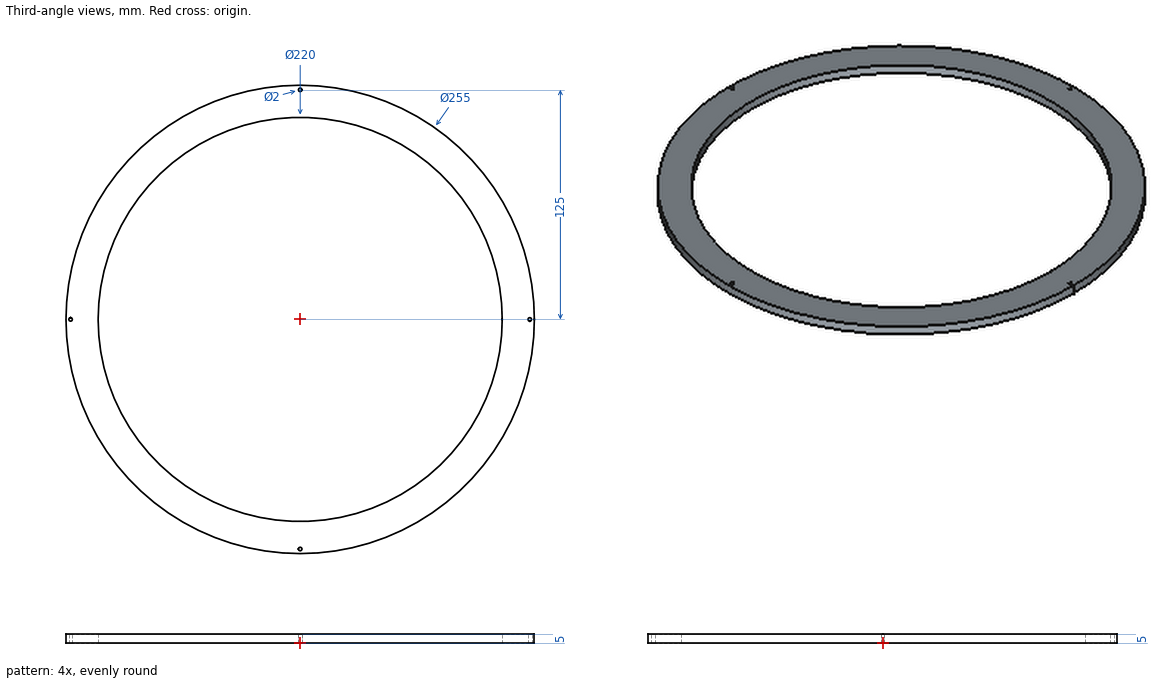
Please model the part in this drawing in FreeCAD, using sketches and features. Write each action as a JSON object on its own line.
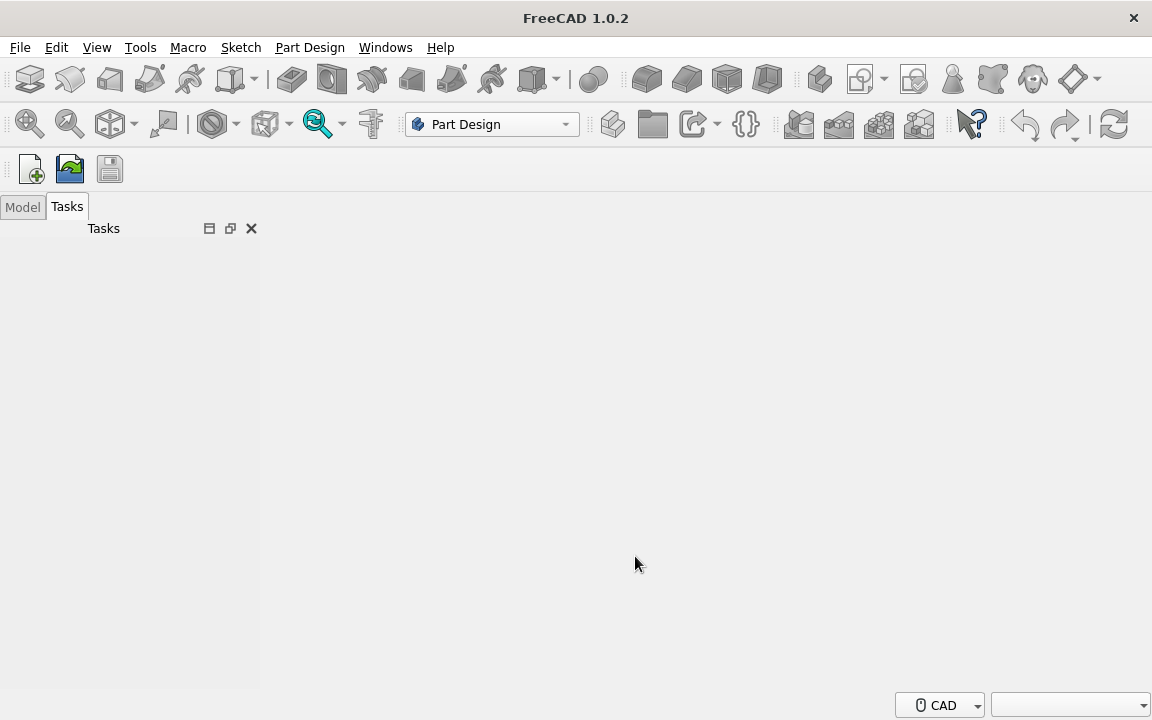
{"action": "left_click", "coordinate": [30, 170]}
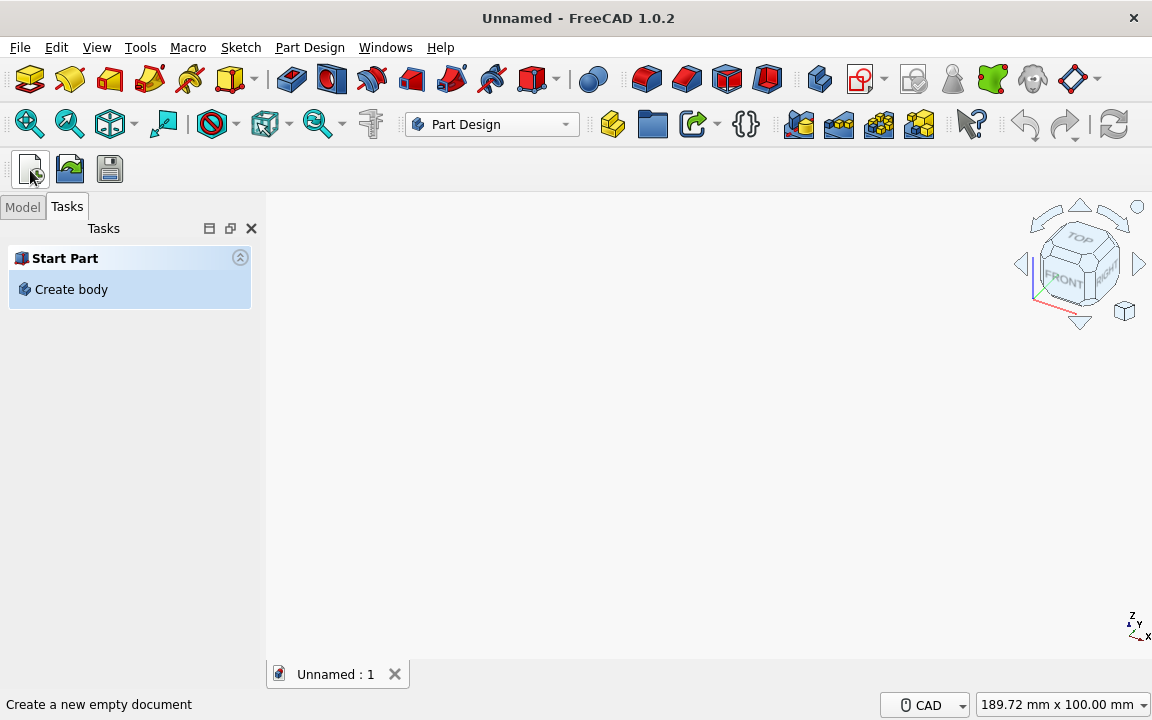
{"action": "left_click", "coordinate": [860, 80]}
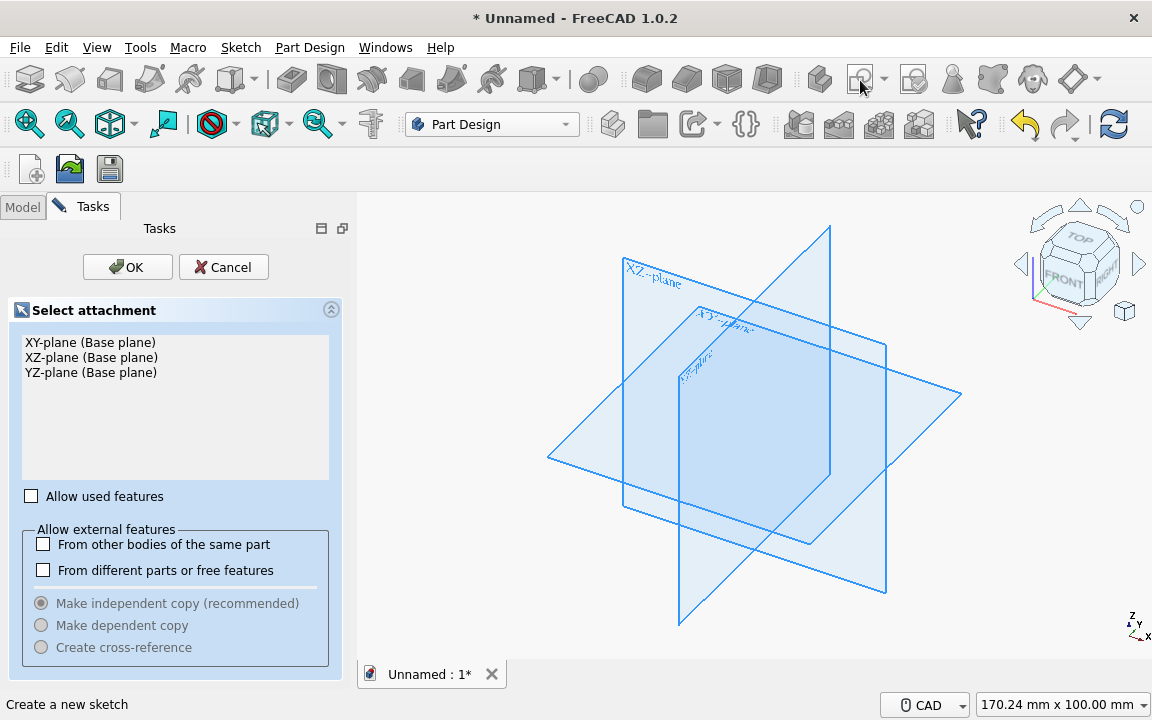
{"action": "left_click", "coordinate": [82, 342]}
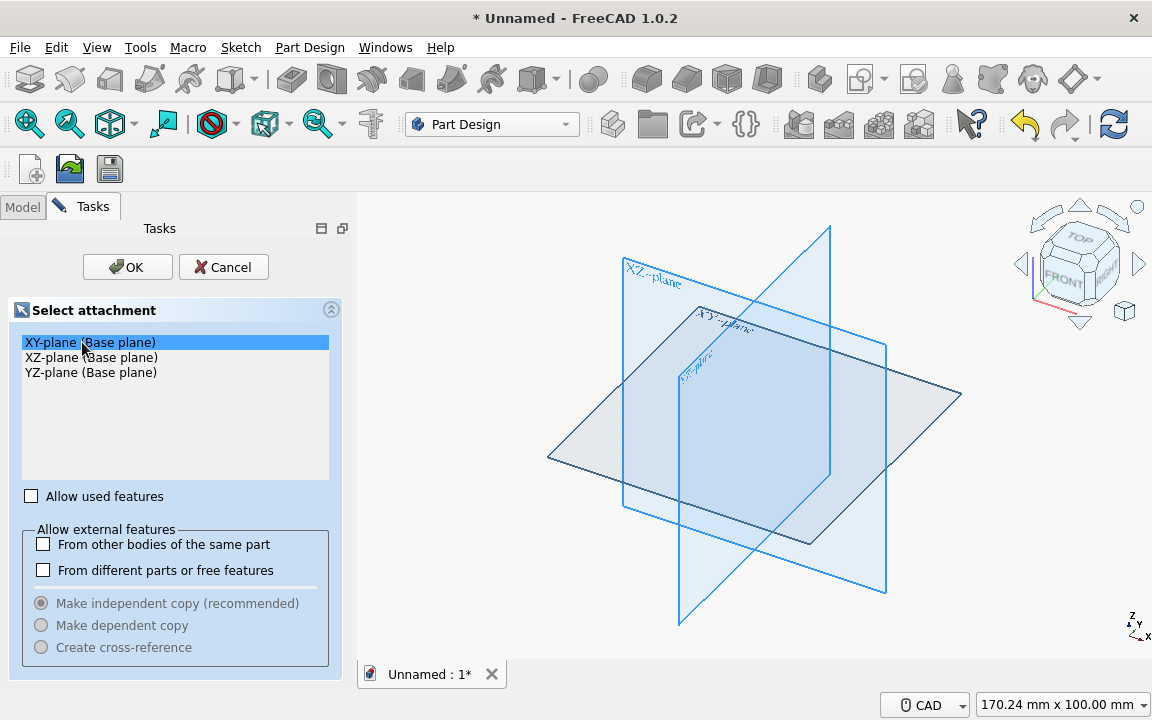
{"action": "left_click", "coordinate": [128, 267]}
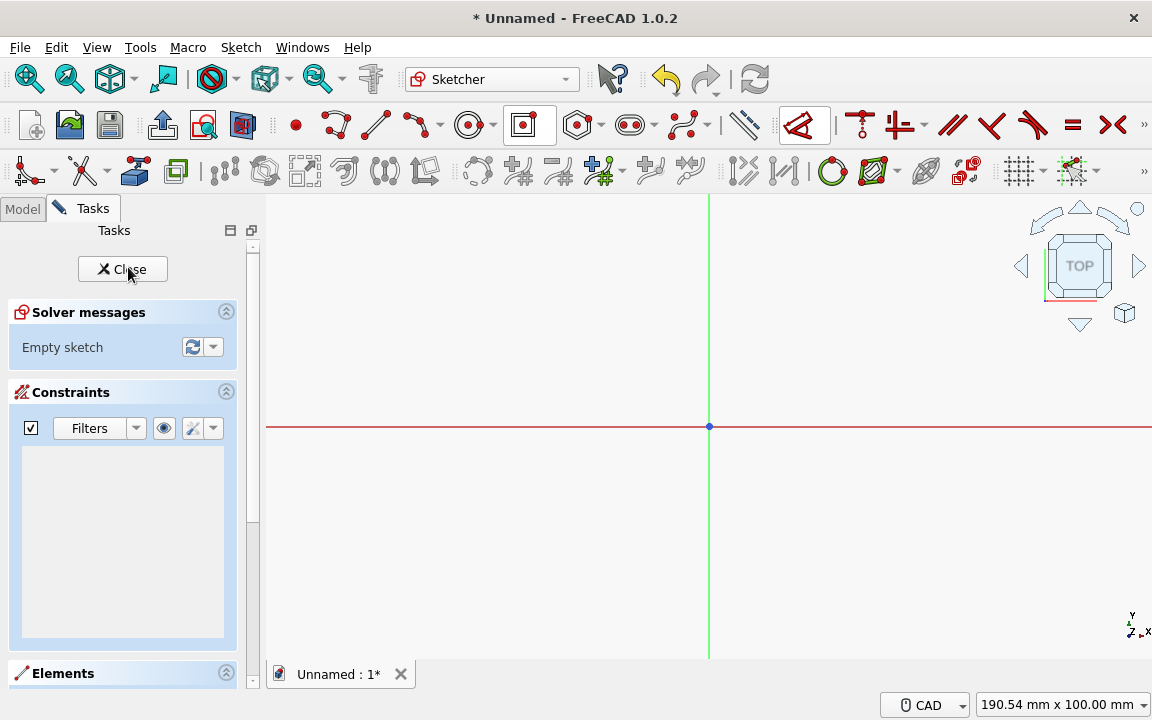
{"action": "scroll", "coordinate": [618, 426], "scroll_direction": "down", "scroll_amount": 7}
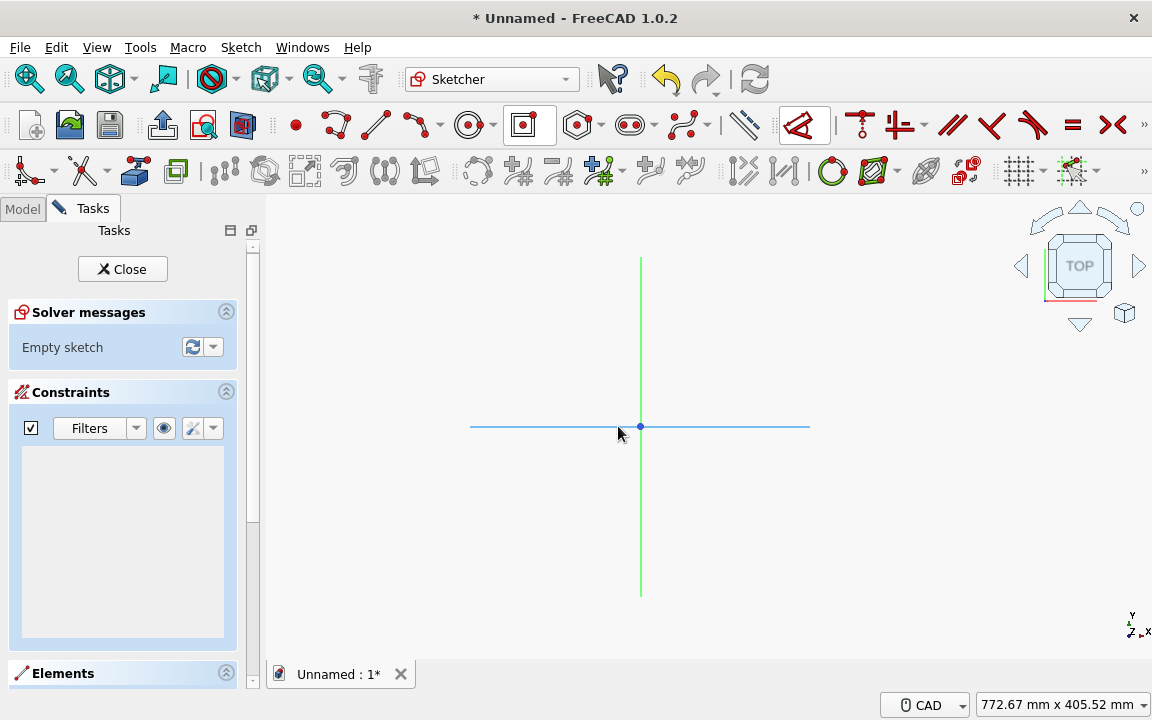
{"action": "left_click", "coordinate": [470, 126]}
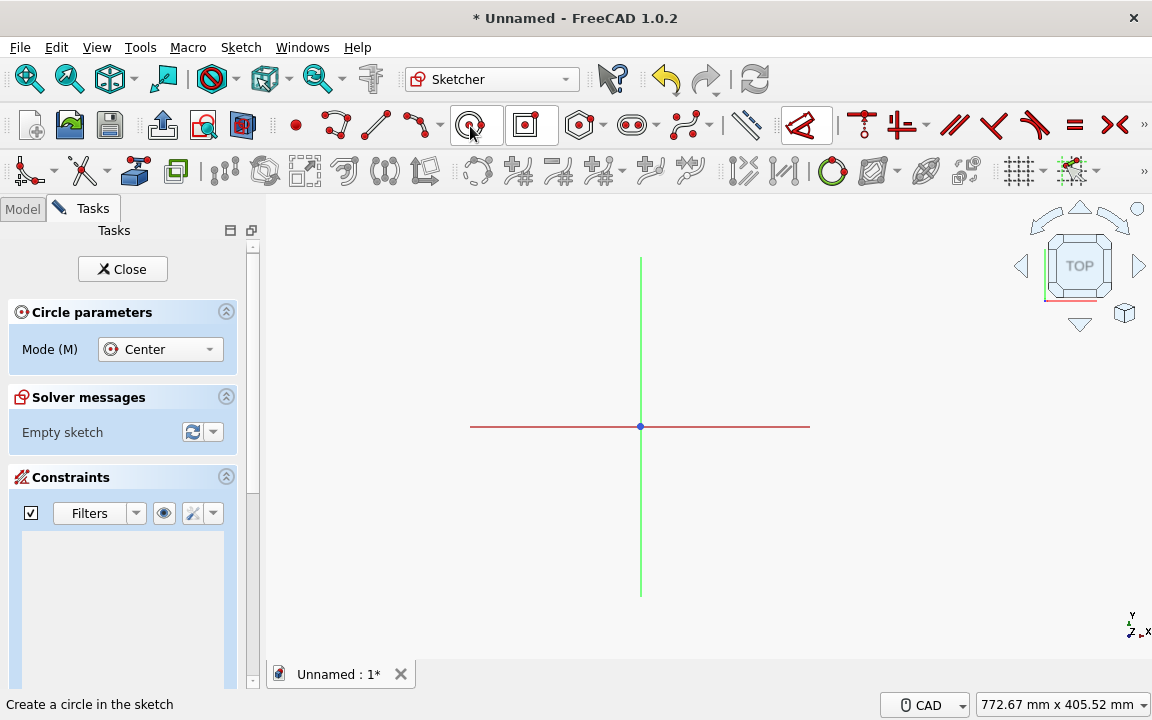
{"action": "left_click", "coordinate": [641, 426]}
{"action": "mouse_move", "coordinate": [744, 323]}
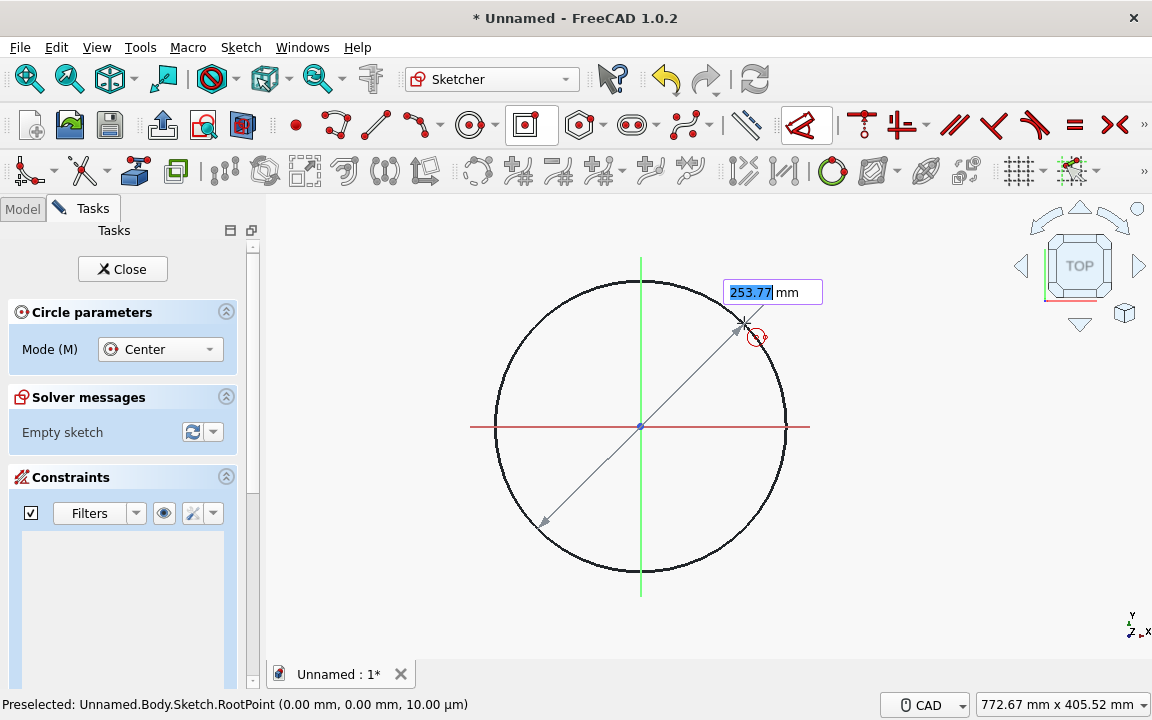
{"action": "type", "text": "255"}
{"action": "key", "text": "Return"}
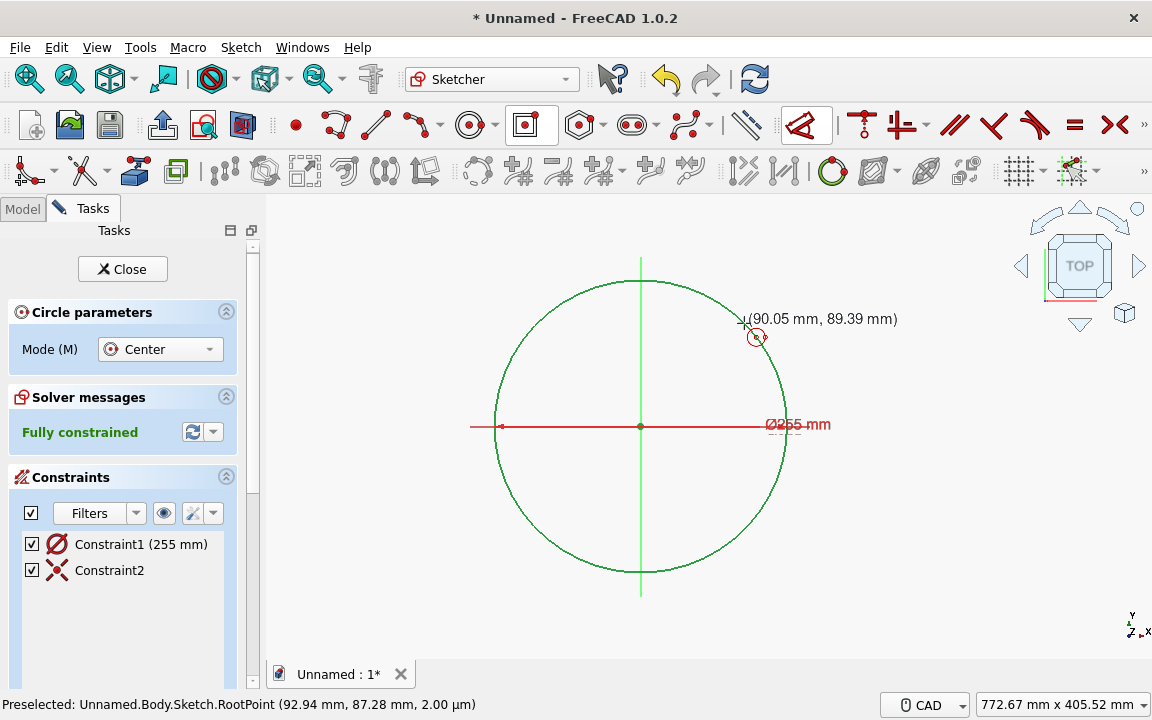
{"action": "left_click", "coordinate": [641, 426]}
{"action": "mouse_move", "coordinate": [730, 337]}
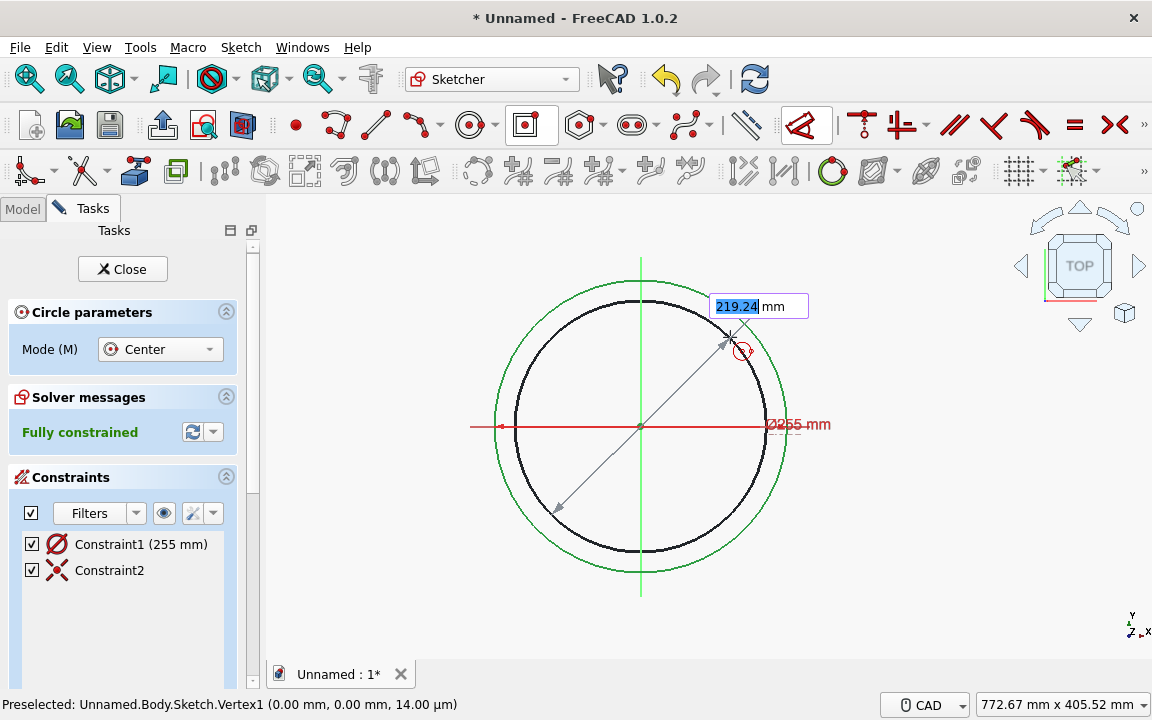
{"action": "type", "text": "220"}
{"action": "key", "text": "Return"}
{"action": "key", "text": "Escape"}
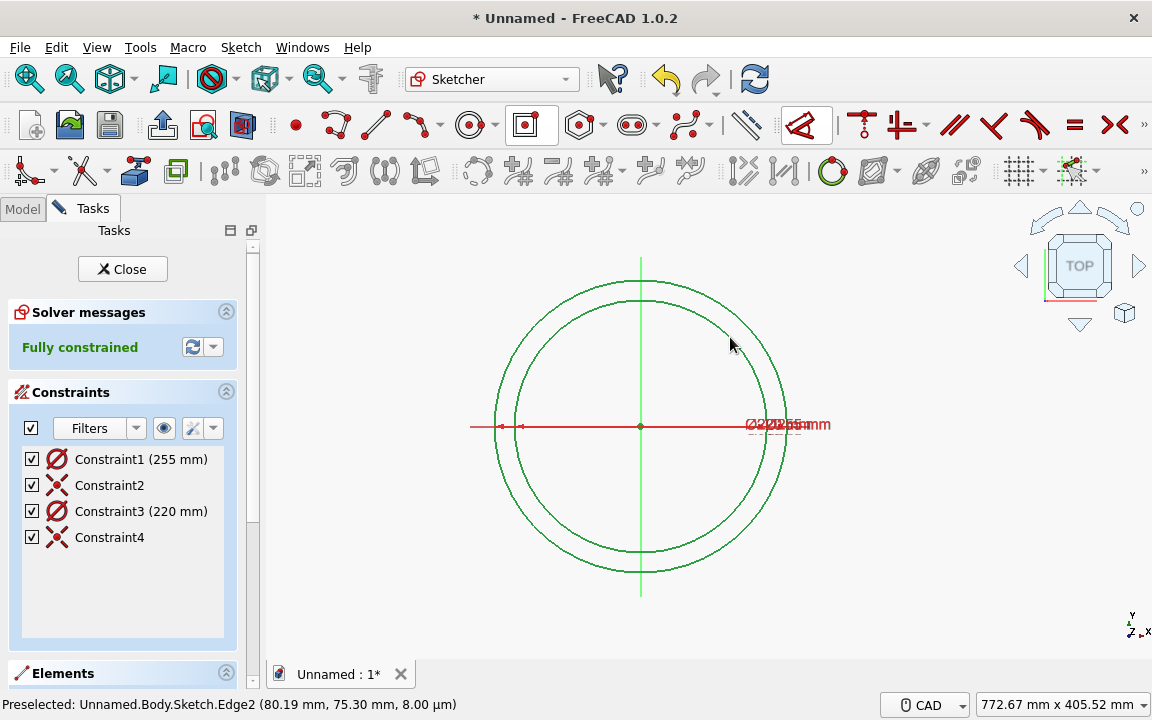
{"action": "left_click", "coordinate": [123, 269]}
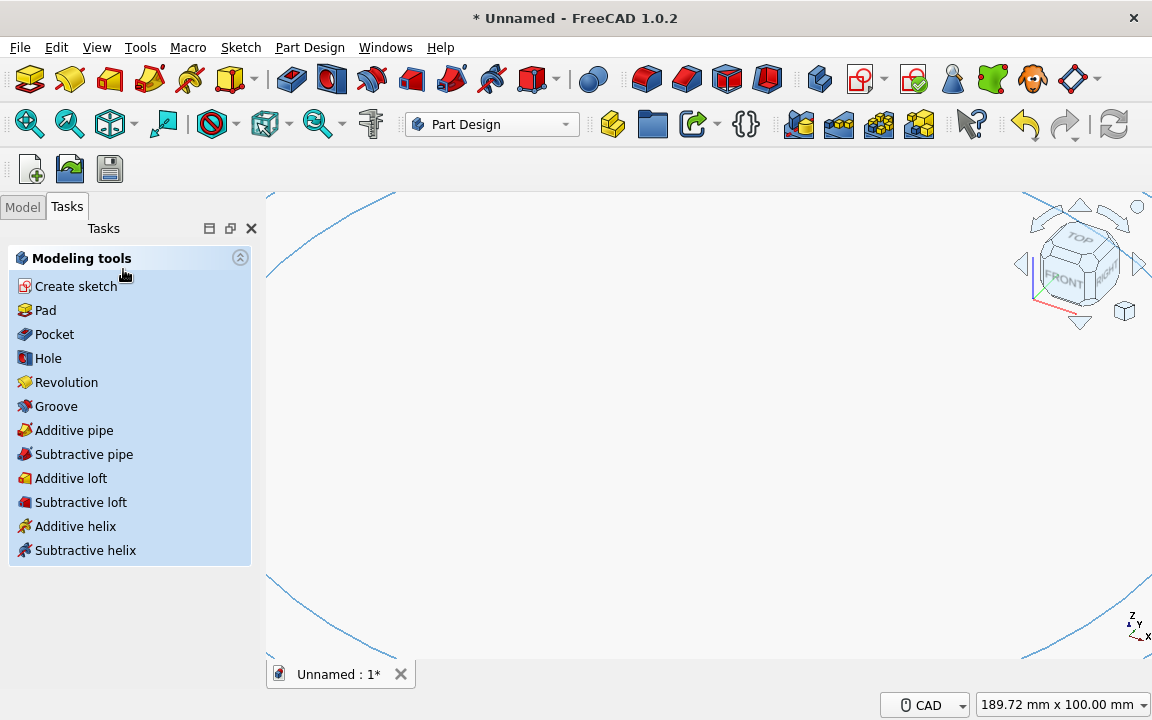
{"action": "left_click", "coordinate": [30, 80]}